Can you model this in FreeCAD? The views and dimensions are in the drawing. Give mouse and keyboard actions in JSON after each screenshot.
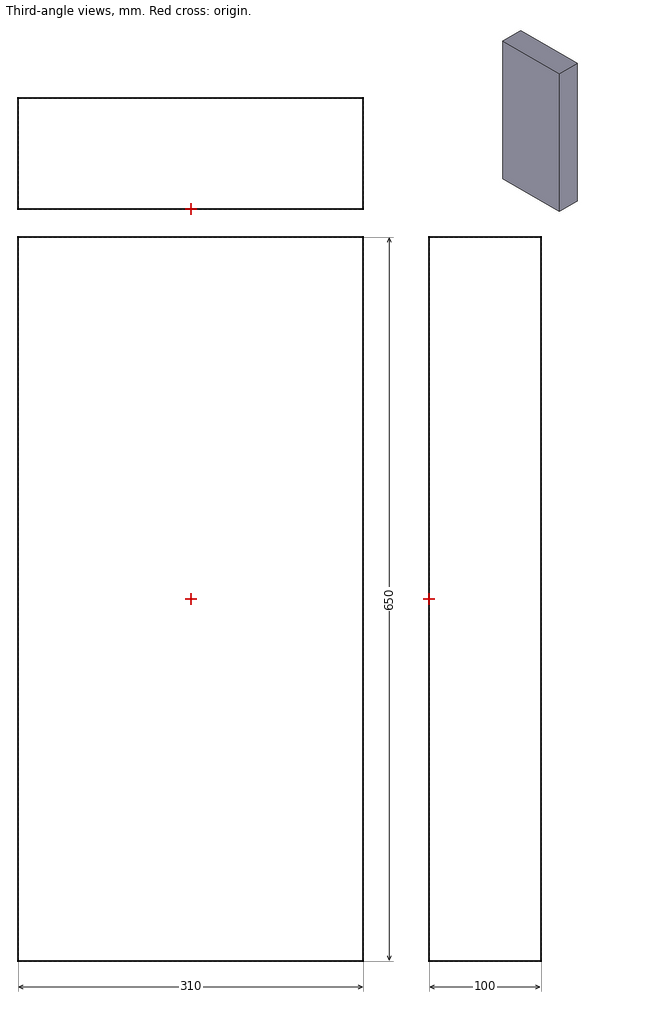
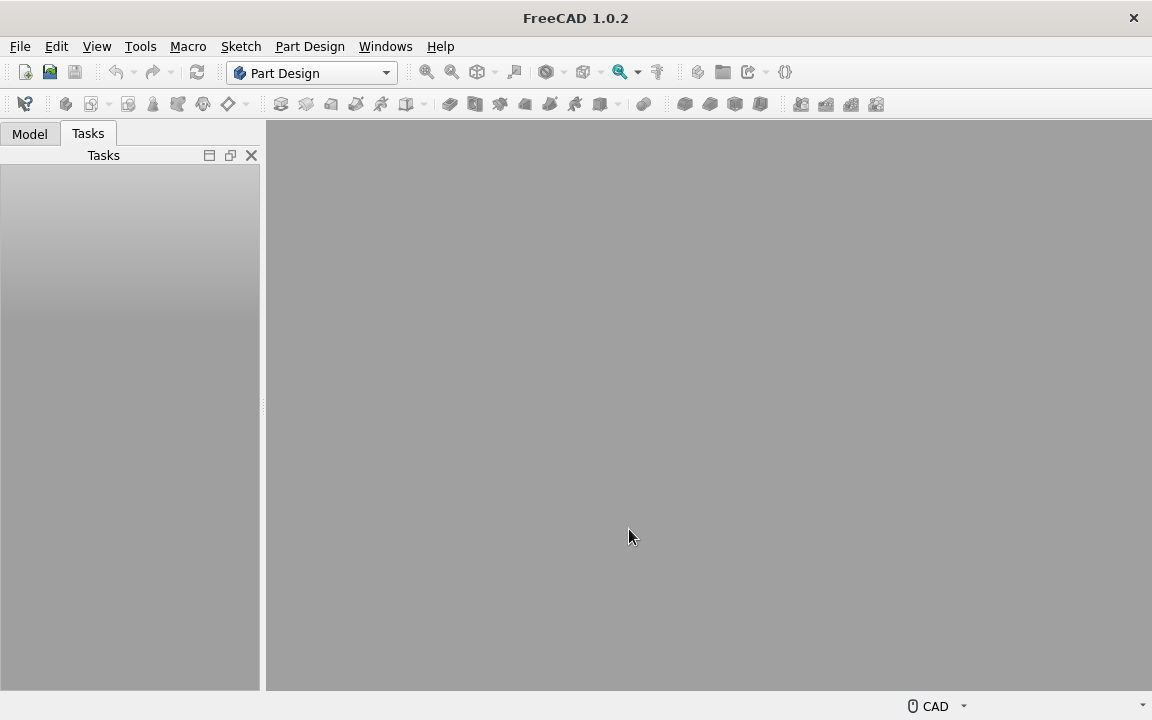
{"action": "left_click", "coordinate": [25, 72]}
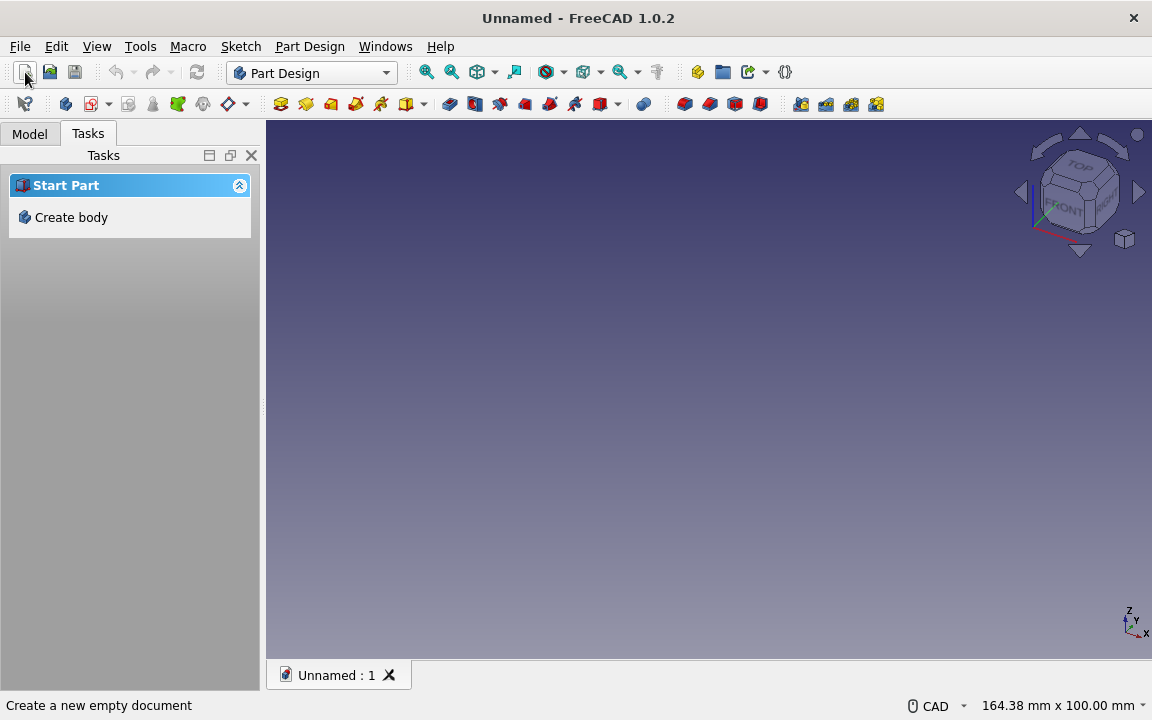
{"action": "left_click", "coordinate": [90, 104]}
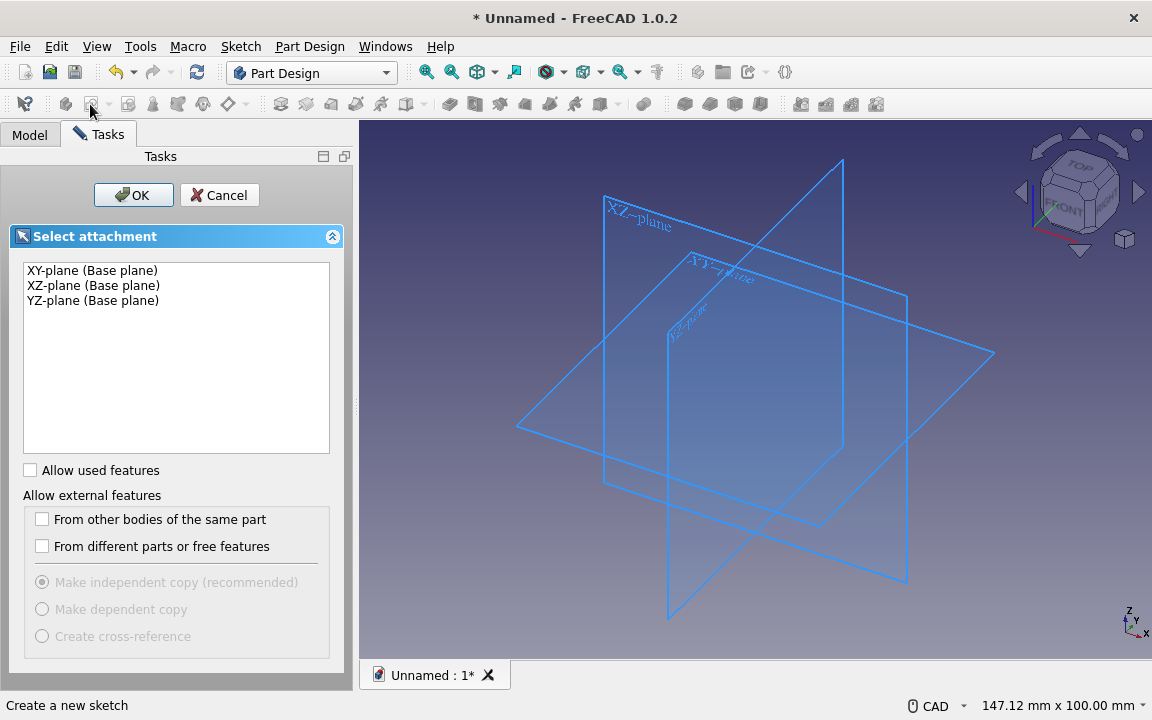
{"action": "left_click", "coordinate": [84, 286]}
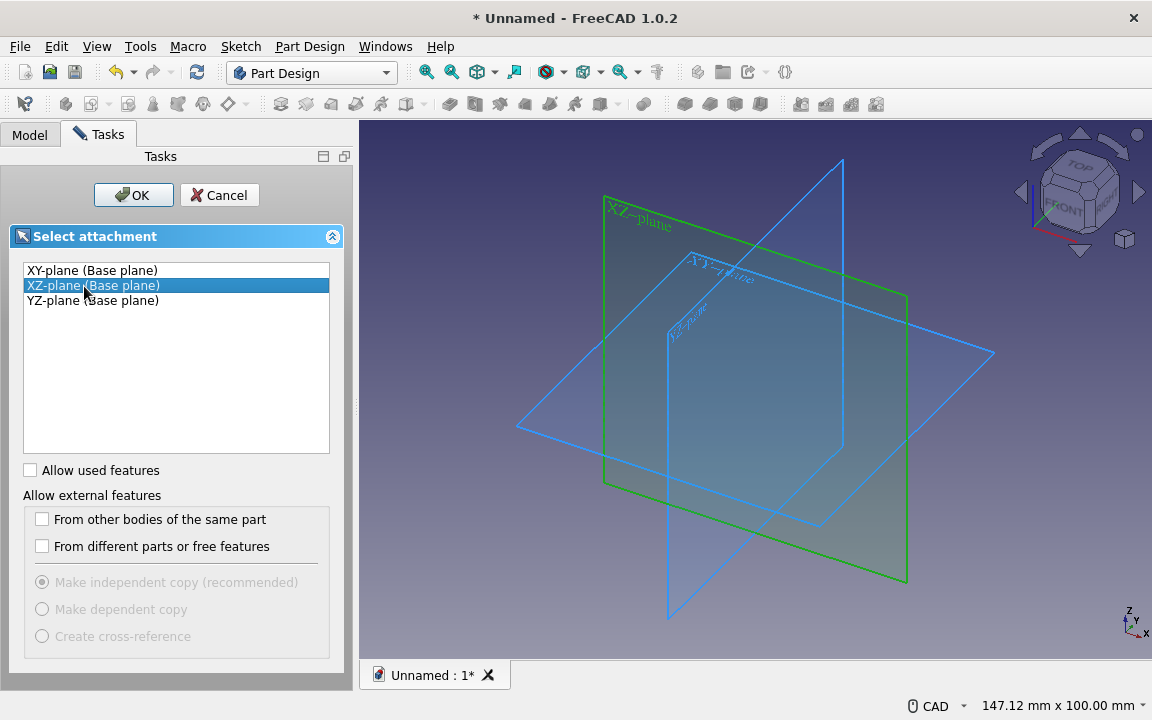
{"action": "left_click", "coordinate": [134, 195]}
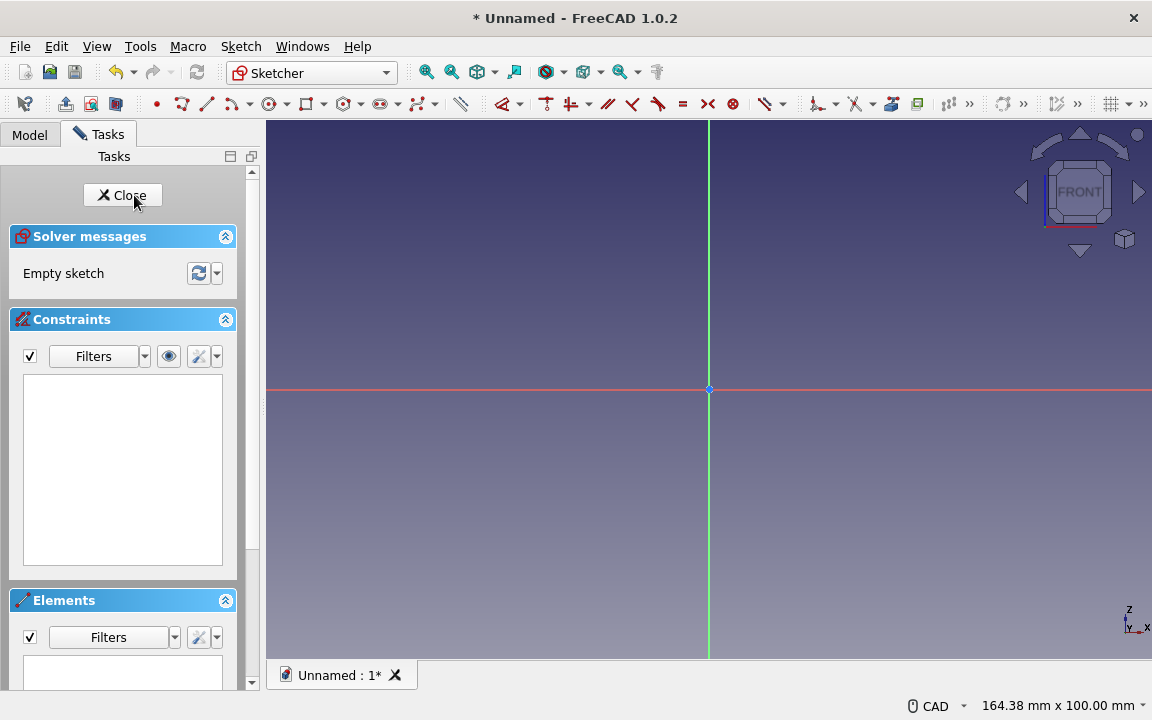
{"action": "scroll", "coordinate": [634, 390], "scroll_direction": "down", "scroll_amount": 12}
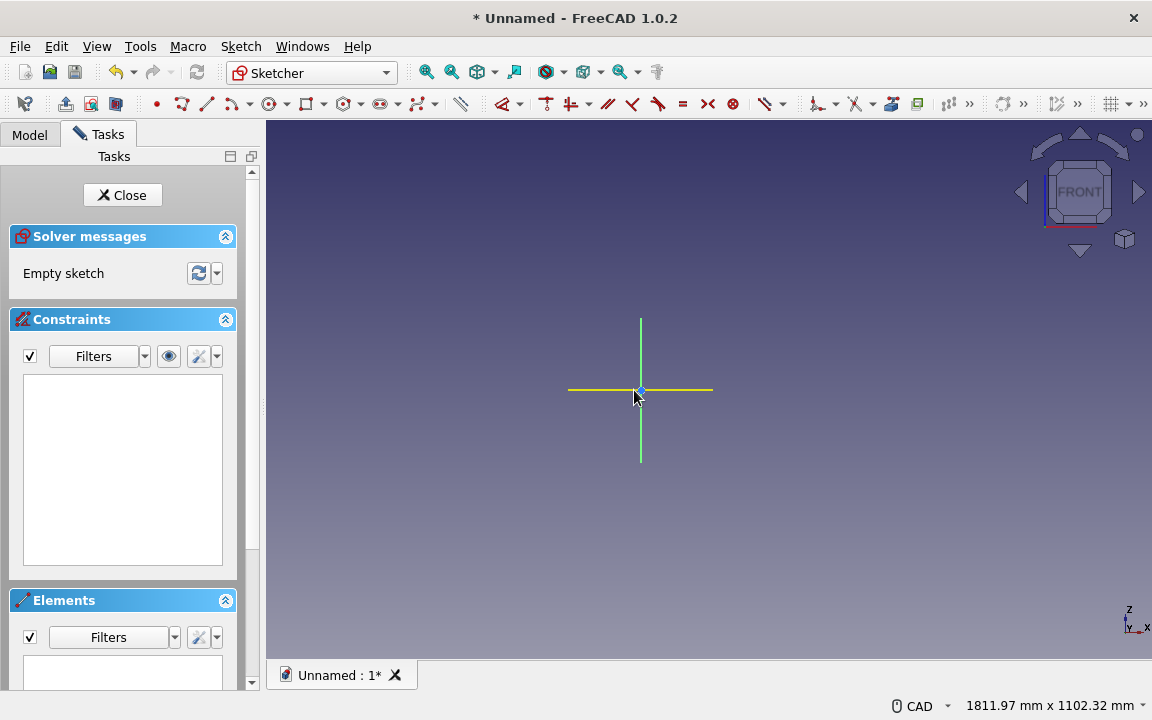
{"action": "key", "text": "g v"}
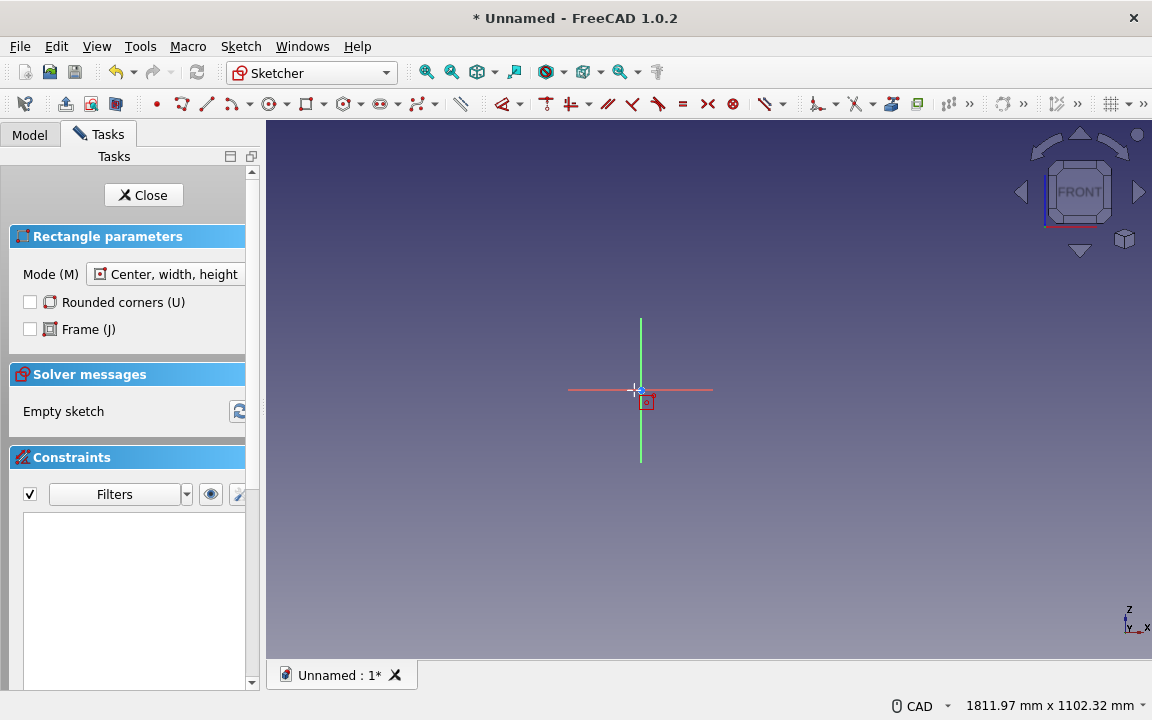
{"action": "left_click", "coordinate": [641, 390]}
{"action": "left_click", "coordinate": [717, 231]}
{"action": "key", "text": "Escape"}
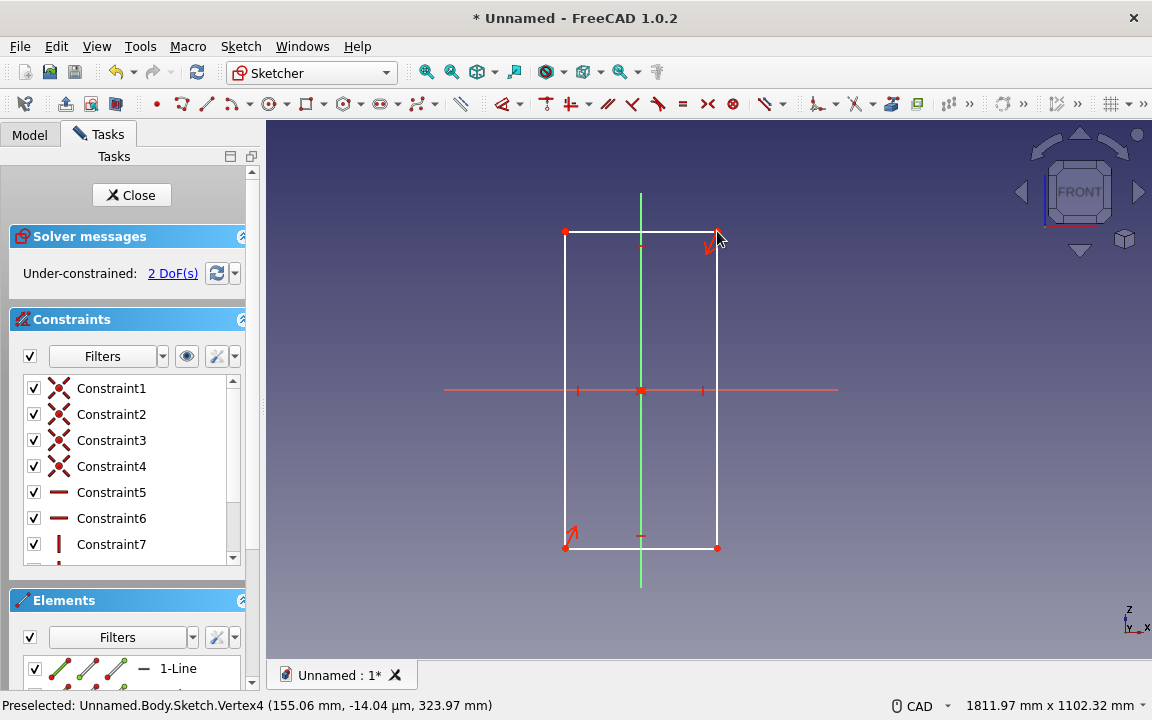
{"action": "left_click", "coordinate": [502, 104]}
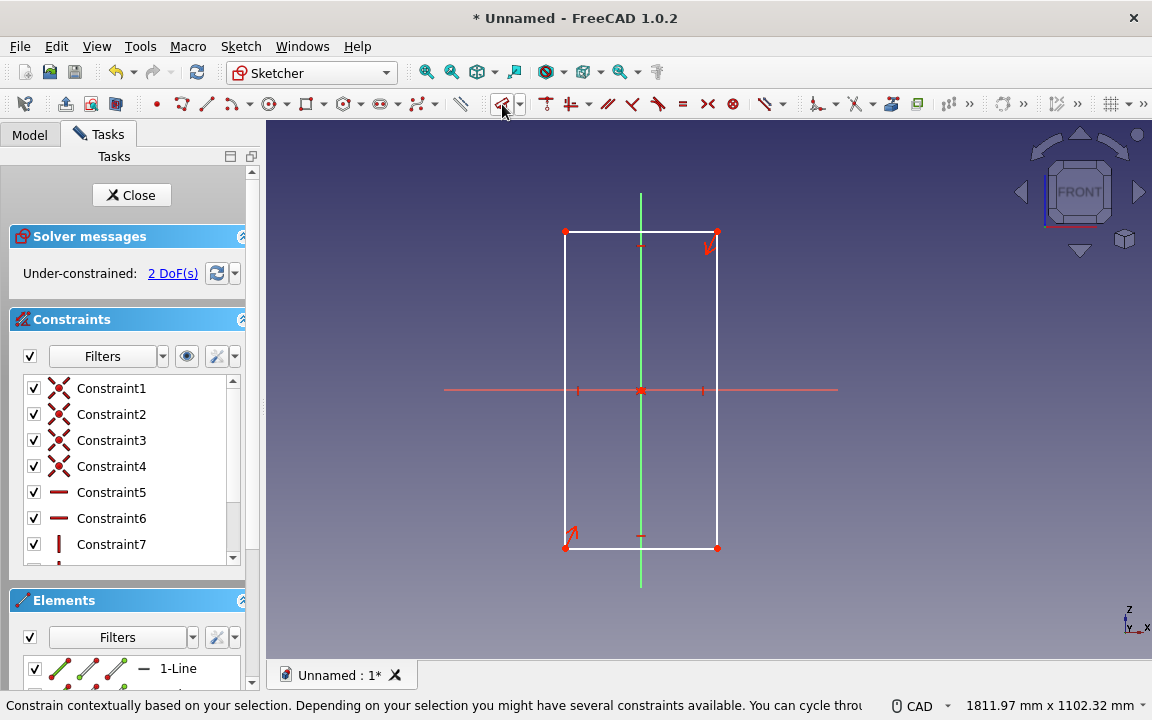
{"action": "left_click", "coordinate": [611, 549]}
{"action": "left_click", "coordinate": [606, 583]}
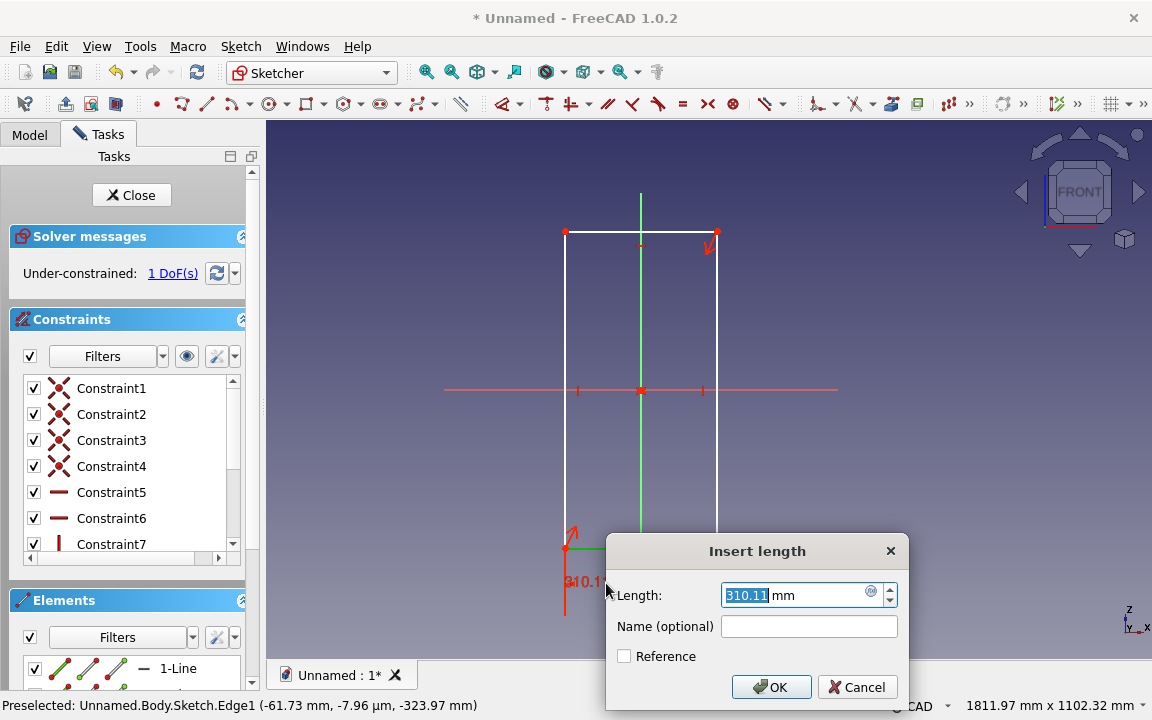
{"action": "type", "text": "310"}
{"action": "key", "text": "Return"}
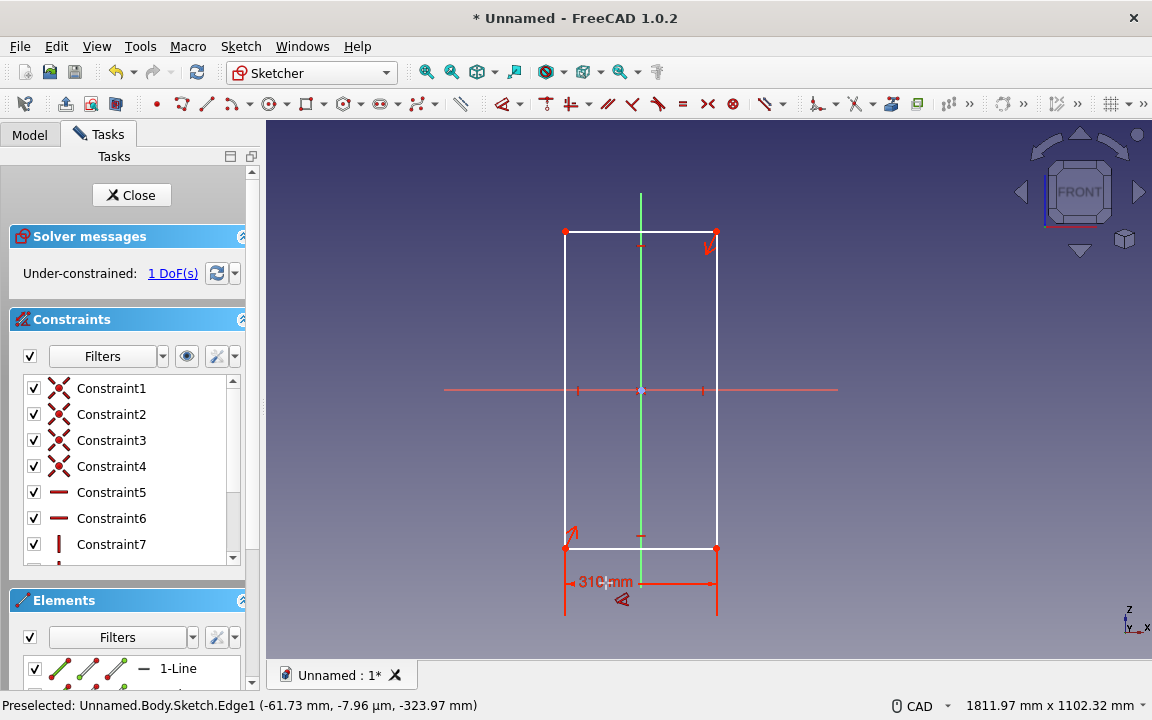
{"action": "left_click", "coordinate": [717, 454]}
{"action": "left_click", "coordinate": [751, 318]}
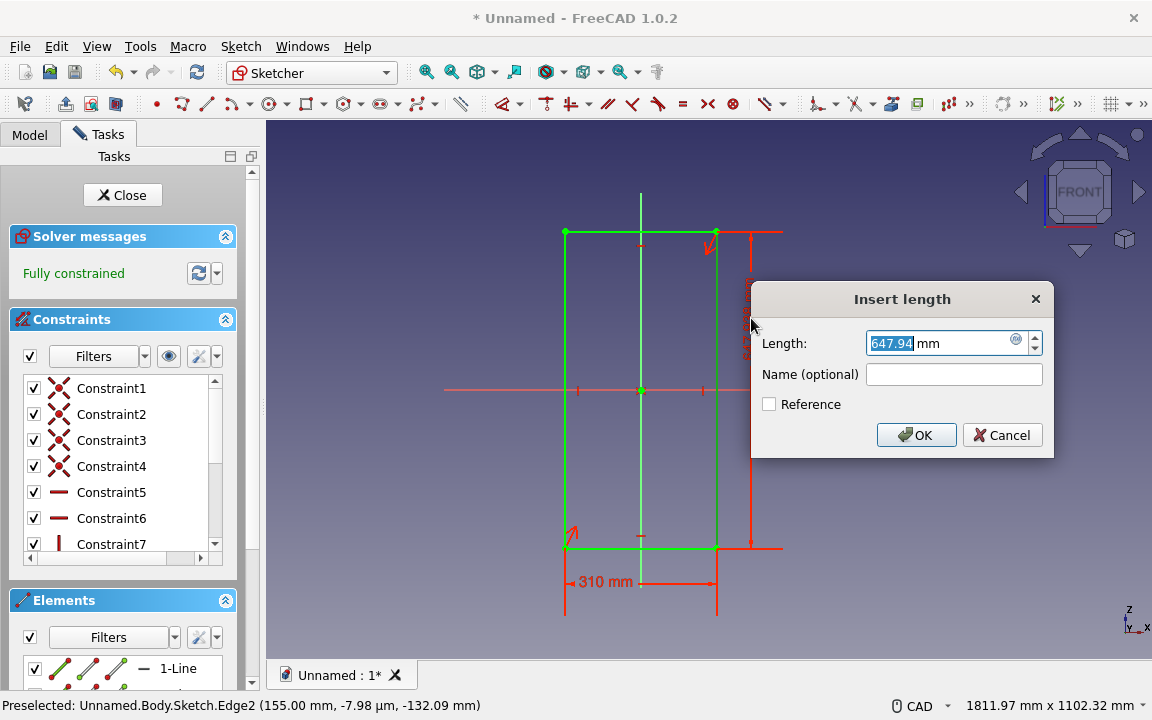
{"action": "type", "text": "650"}
{"action": "key", "text": "Return"}
{"action": "key", "text": "Escape"}